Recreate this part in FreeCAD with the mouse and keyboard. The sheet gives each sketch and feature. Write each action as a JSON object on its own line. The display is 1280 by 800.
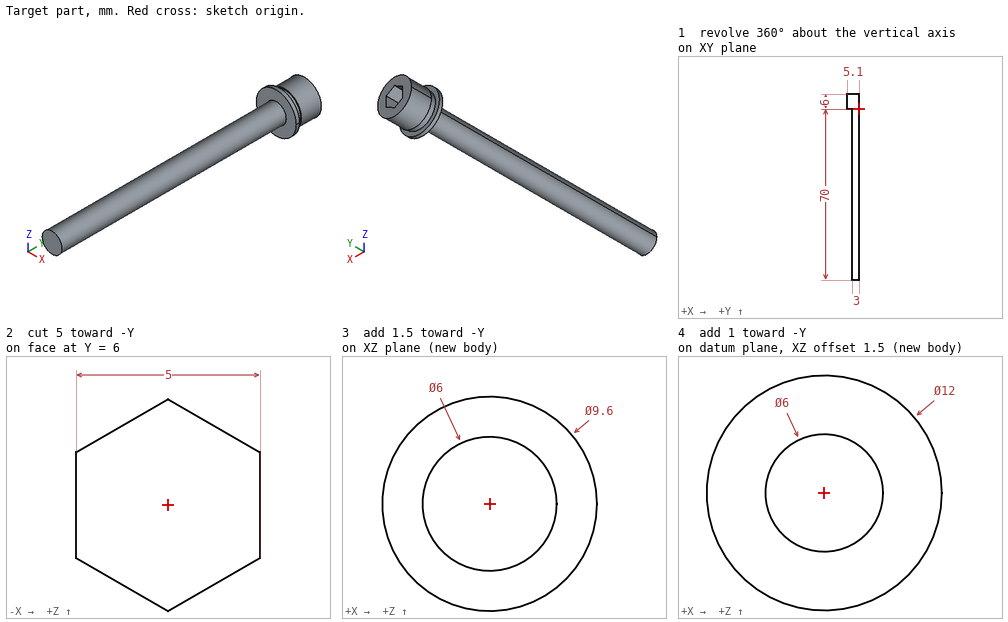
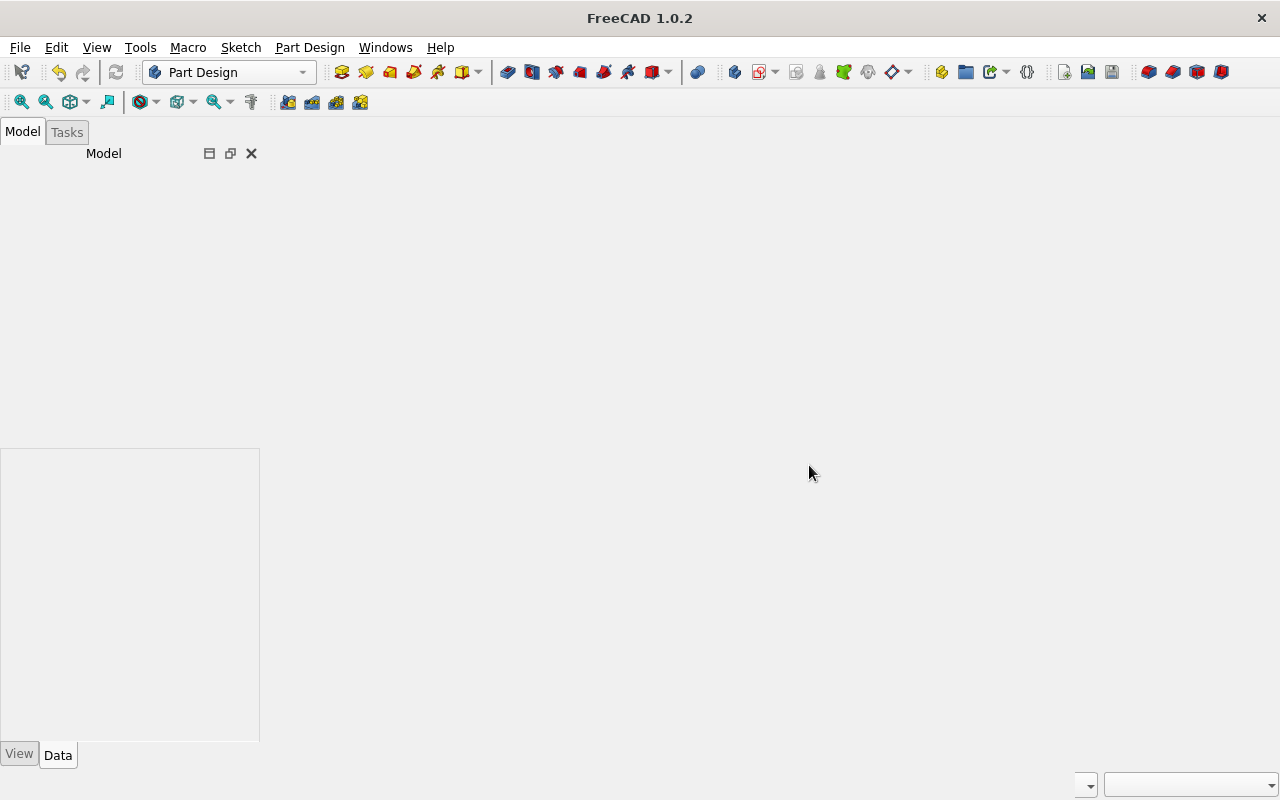
{"action": "left_click", "coordinate": [1064, 72]}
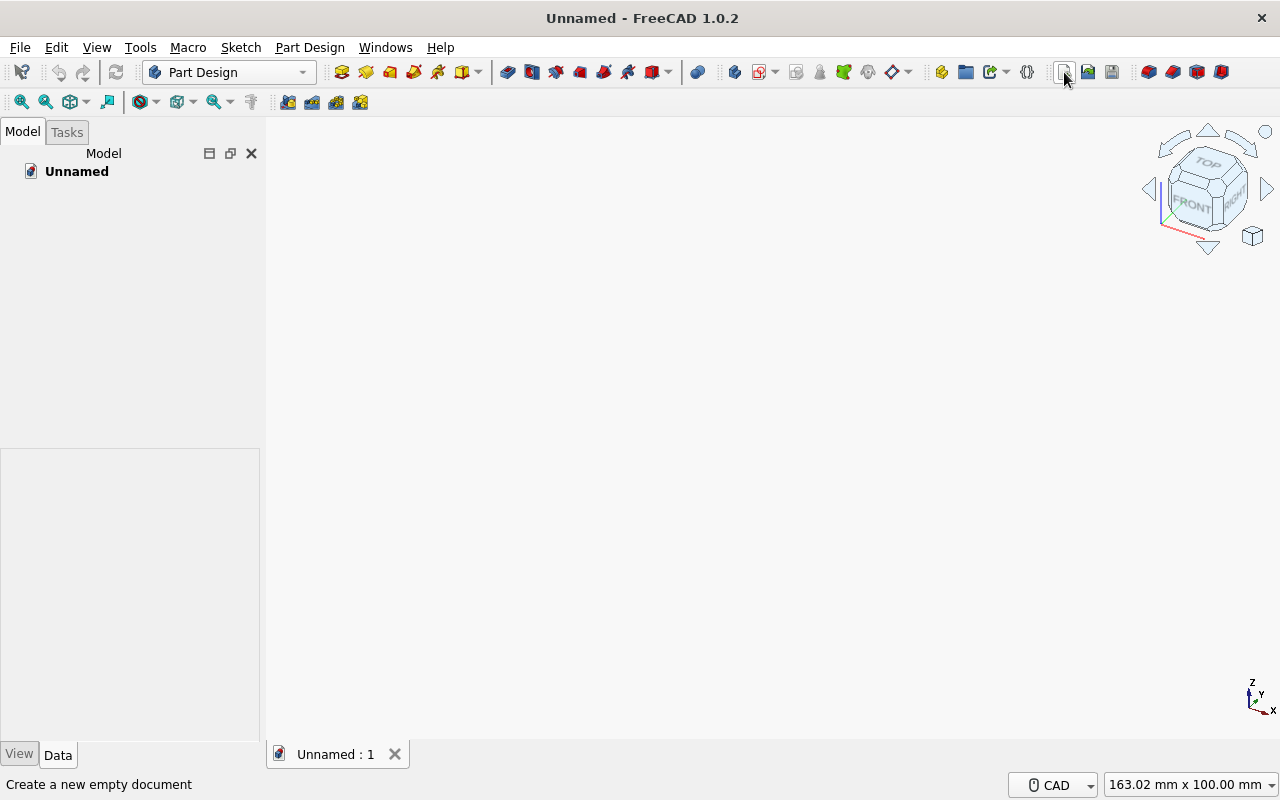
{"action": "left_click", "coordinate": [760, 72]}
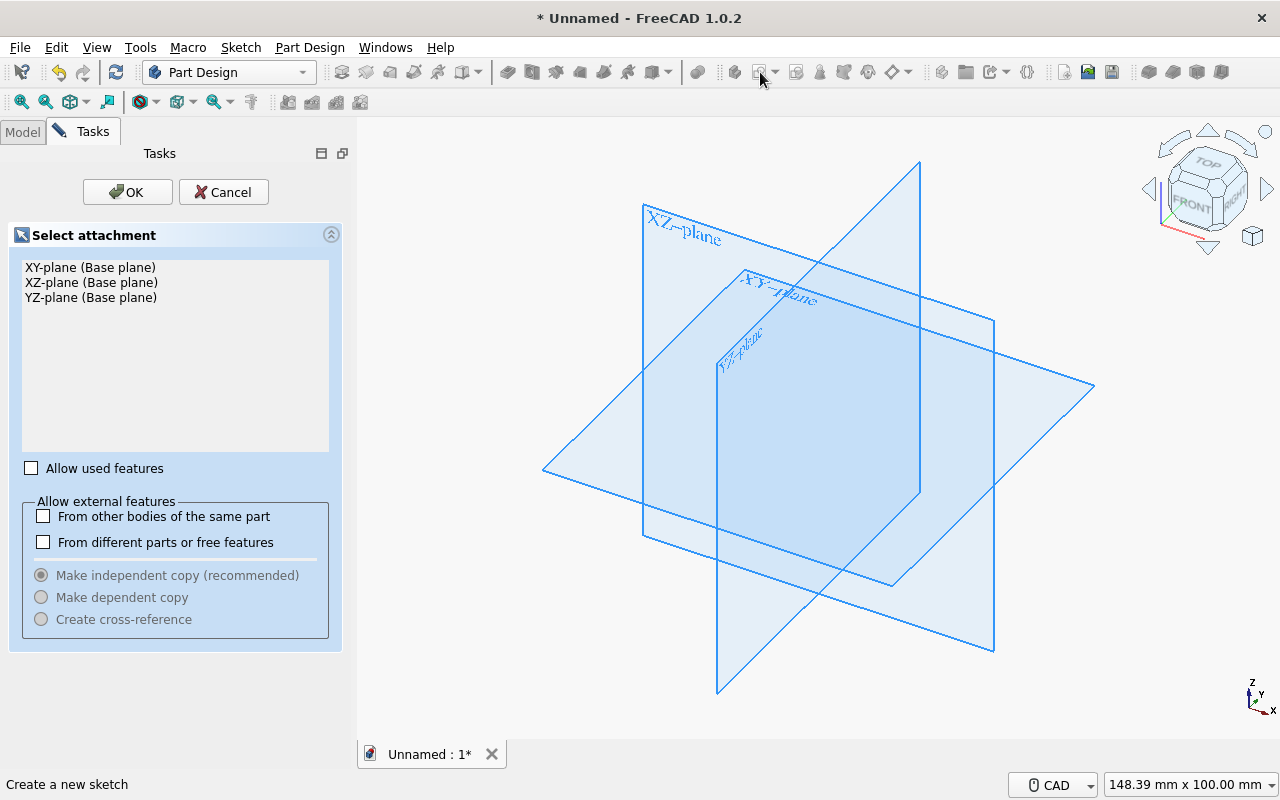
{"action": "left_click", "coordinate": [82, 268]}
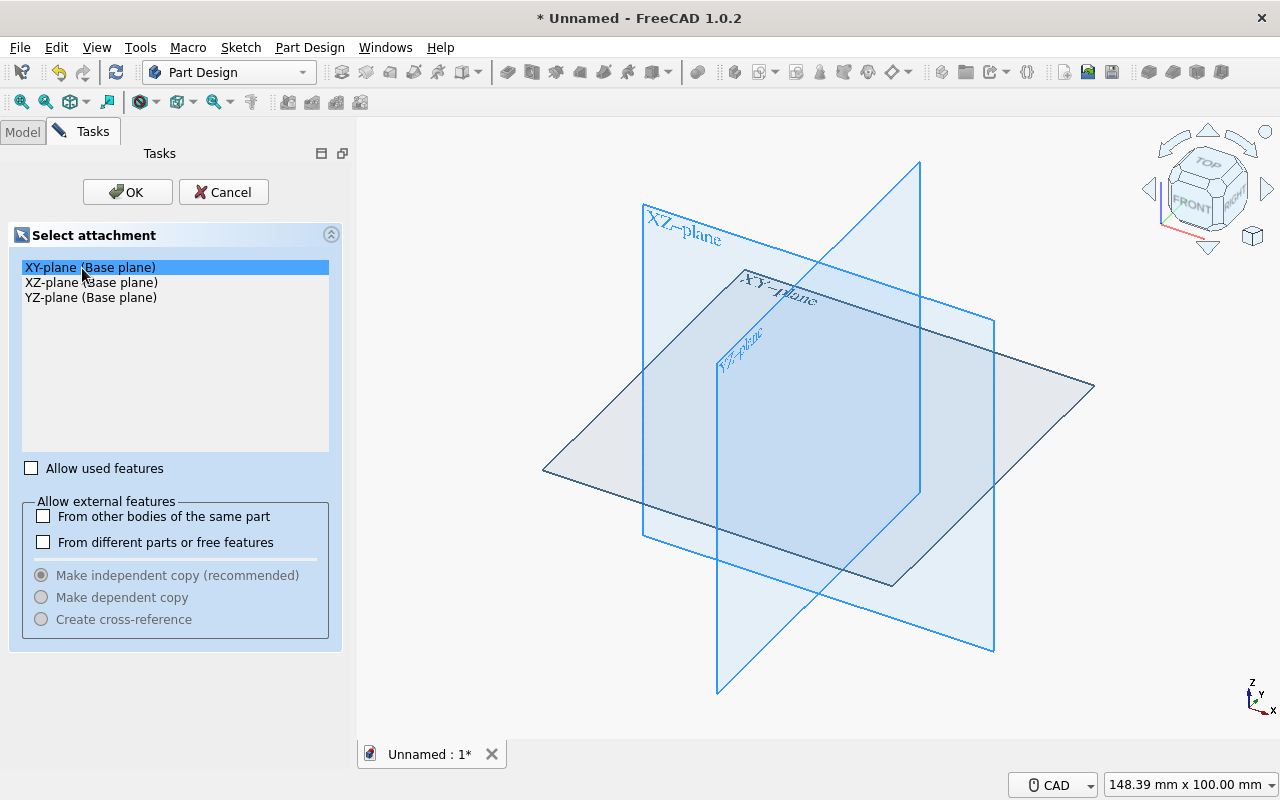
{"action": "left_click", "coordinate": [128, 192]}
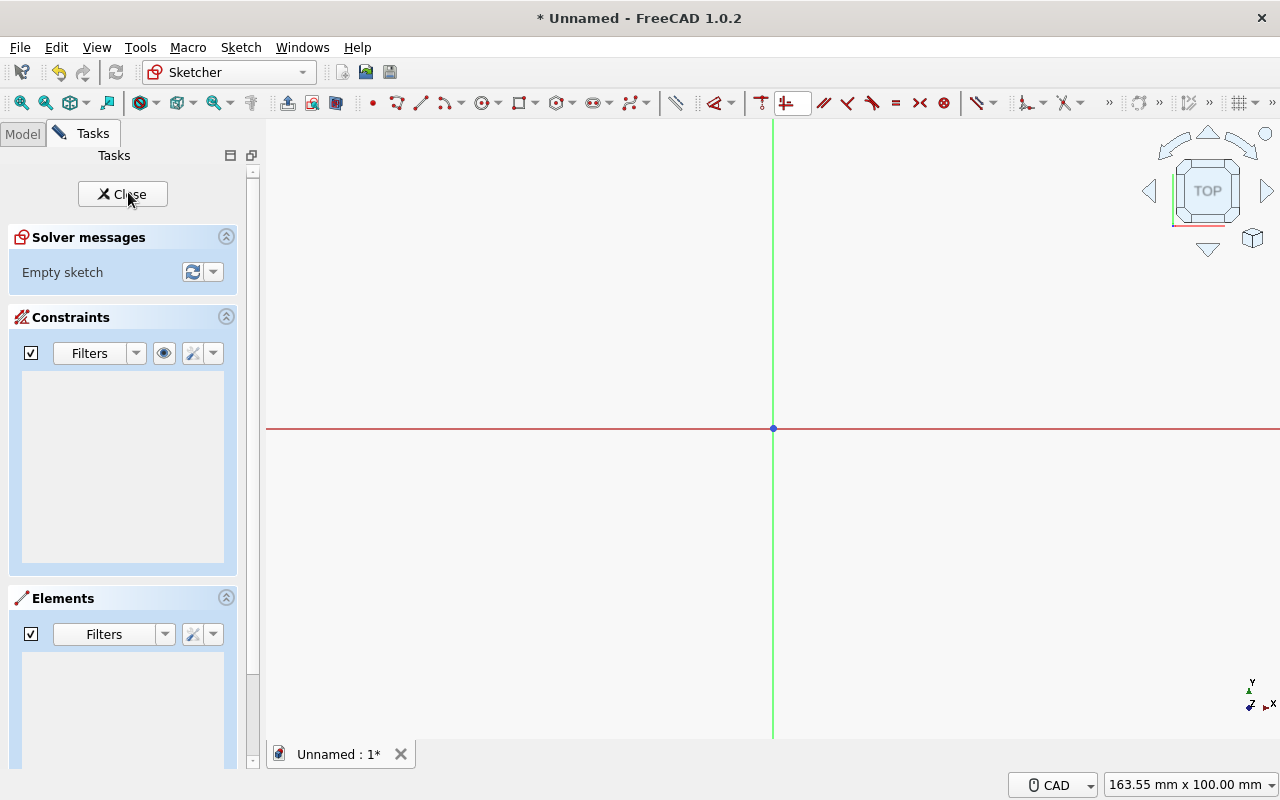
{"action": "scroll", "coordinate": [597, 147], "scroll_direction": "down", "scroll_amount": 2}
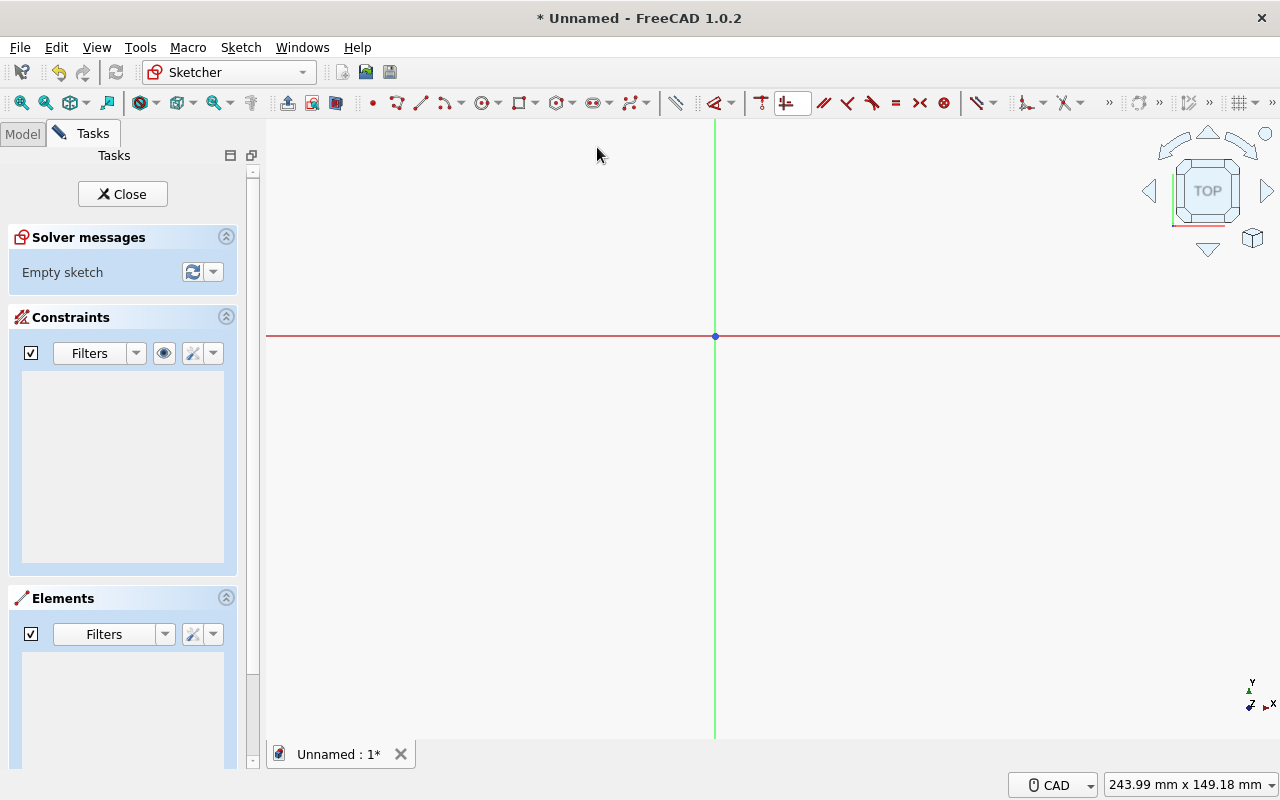
{"action": "left_click", "coordinate": [398, 104]}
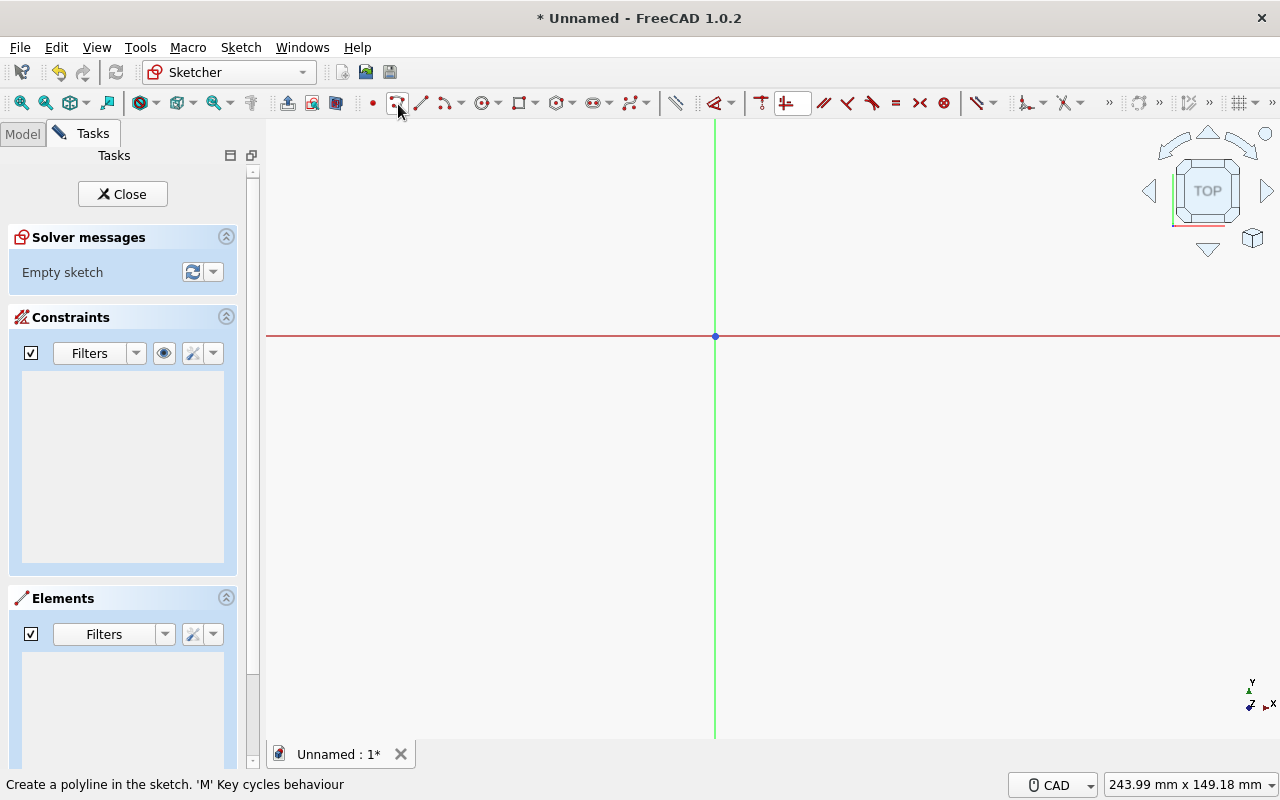
{"action": "scroll", "coordinate": [703, 336], "scroll_direction": "up", "scroll_amount": 2}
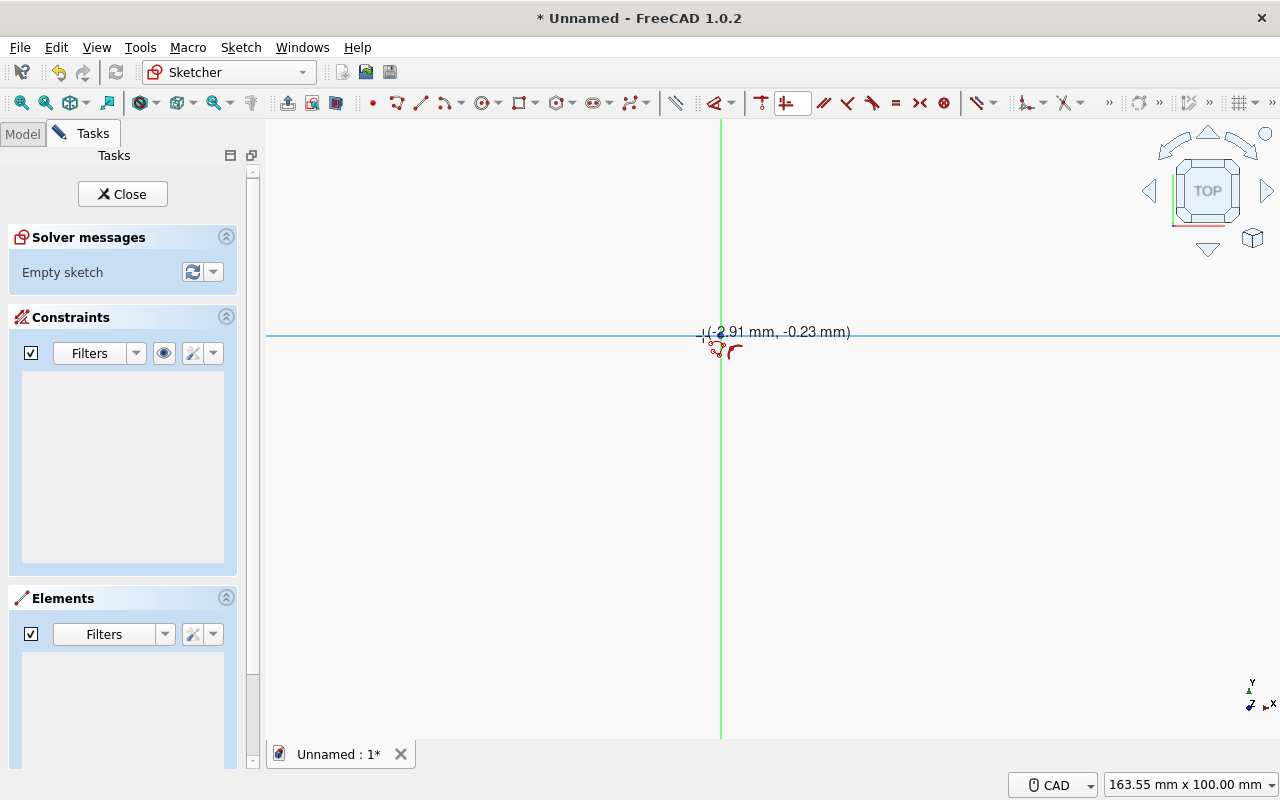
{"action": "left_click", "coordinate": [702, 336]}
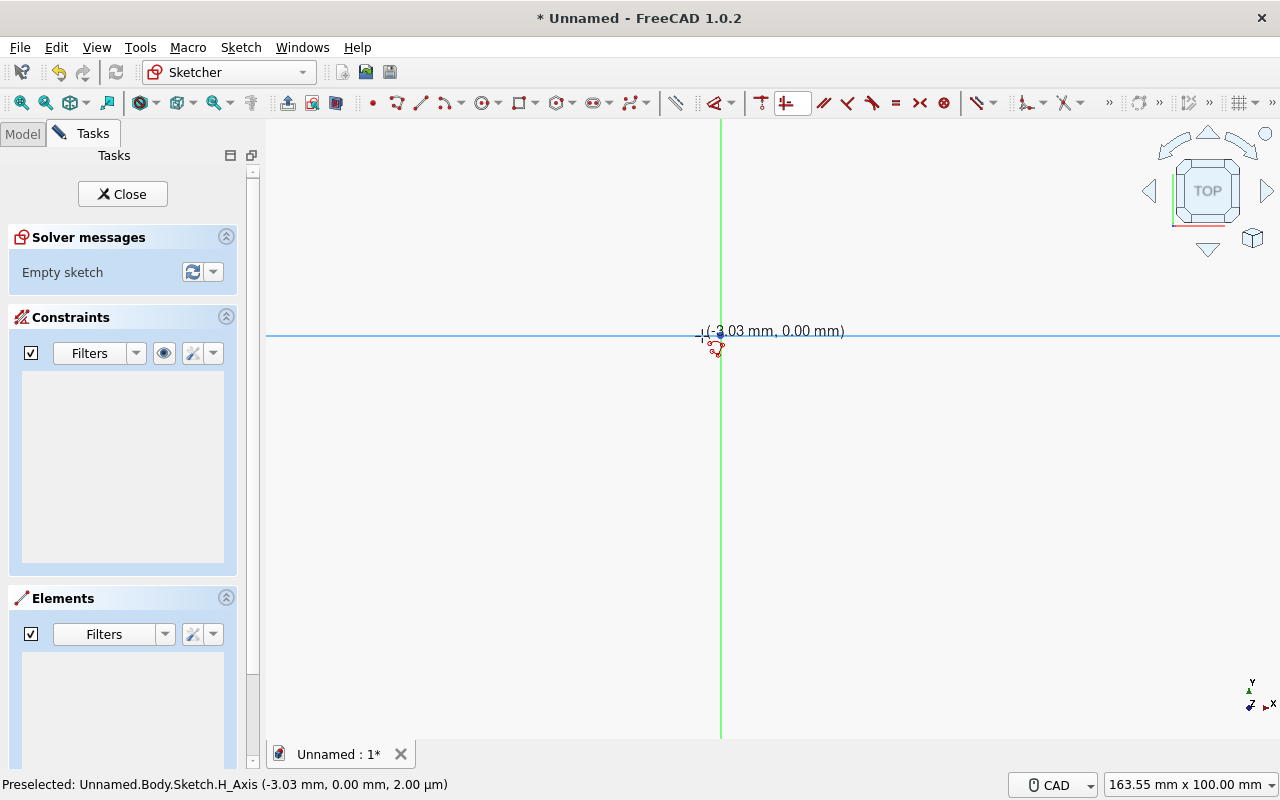
{"action": "scroll", "coordinate": [702, 147], "scroll_direction": "down", "scroll_amount": 1}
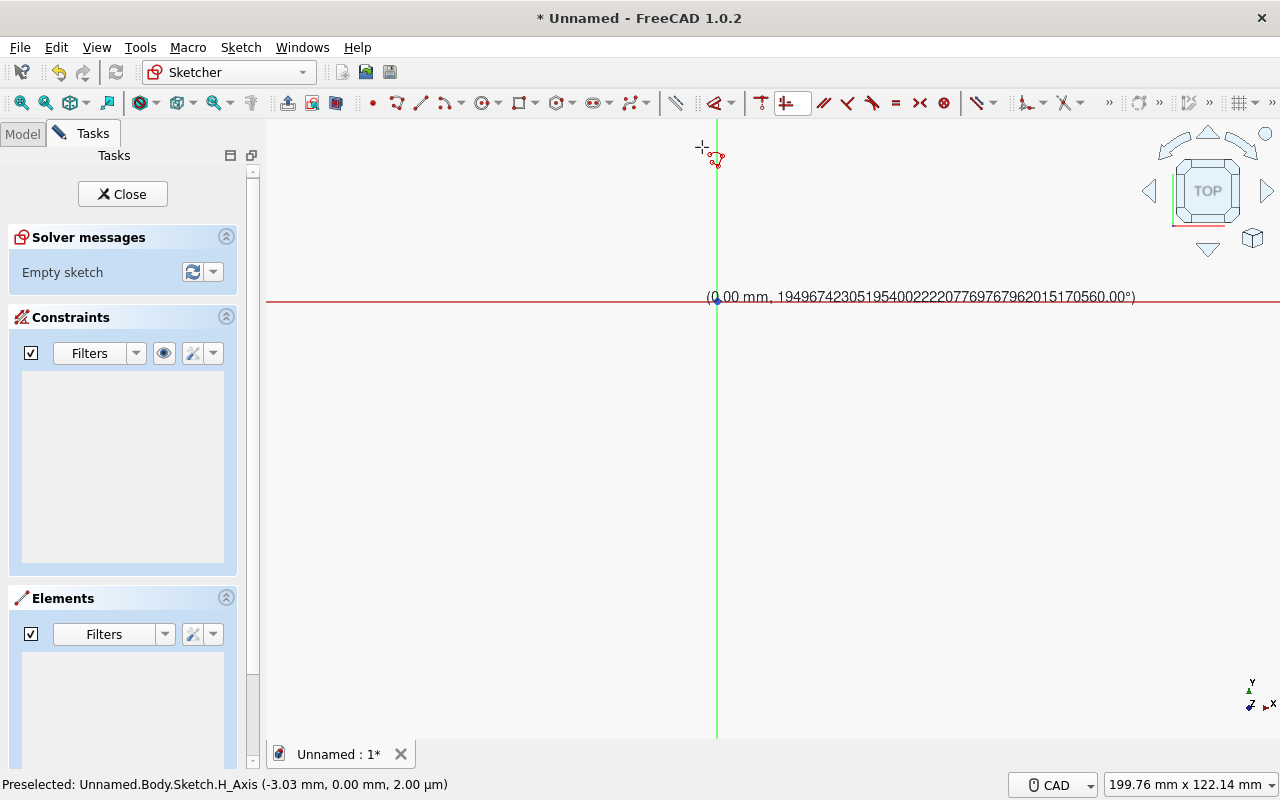
{"action": "left_click", "coordinate": [702, 657]}
{"action": "left_click", "coordinate": [717, 657]}
{"action": "left_click", "coordinate": [708, 271]}
{"action": "left_click", "coordinate": [692, 271]}